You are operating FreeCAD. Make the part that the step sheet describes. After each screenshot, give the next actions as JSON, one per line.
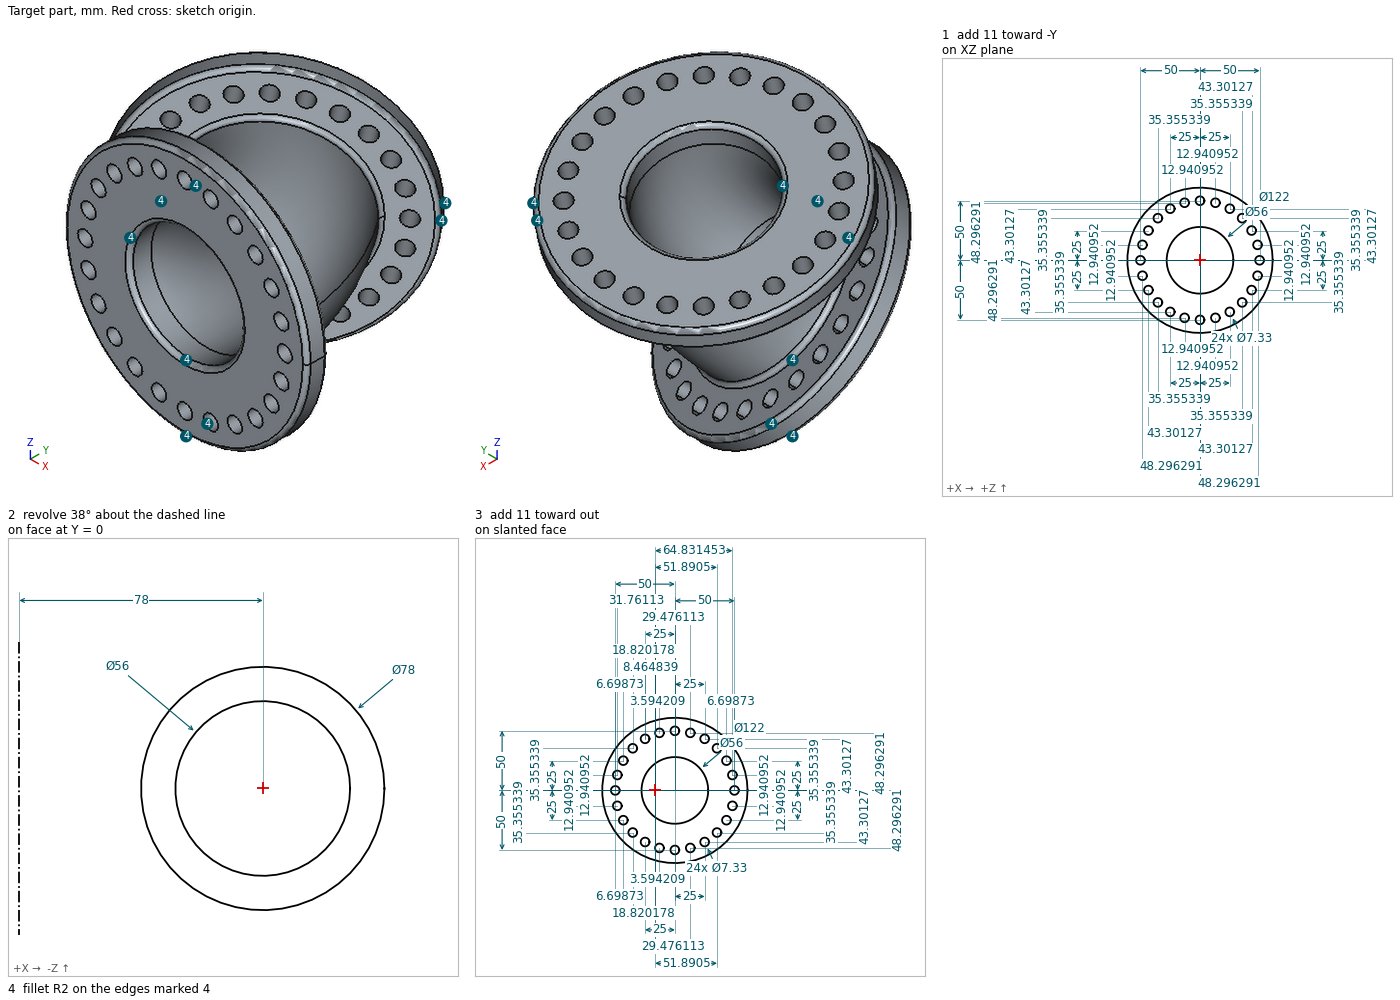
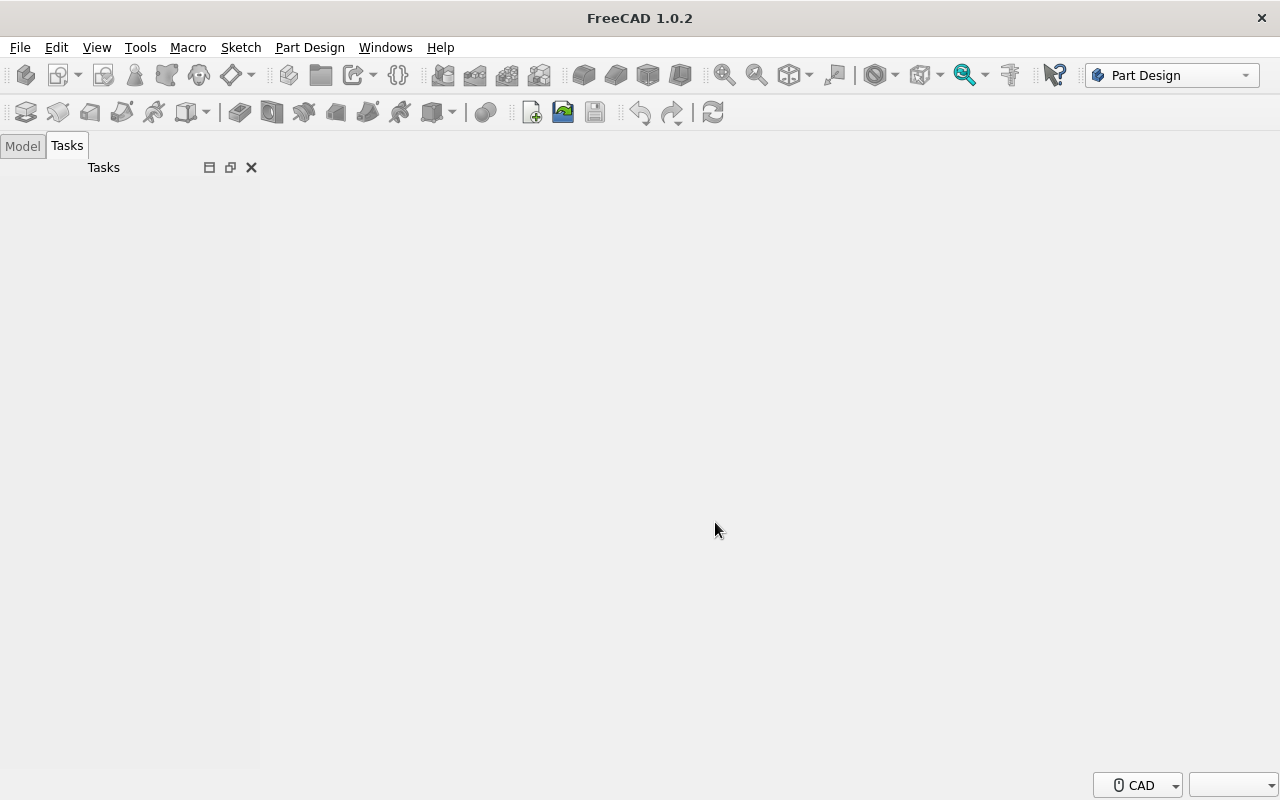
{"action": "left_click", "coordinate": [532, 112]}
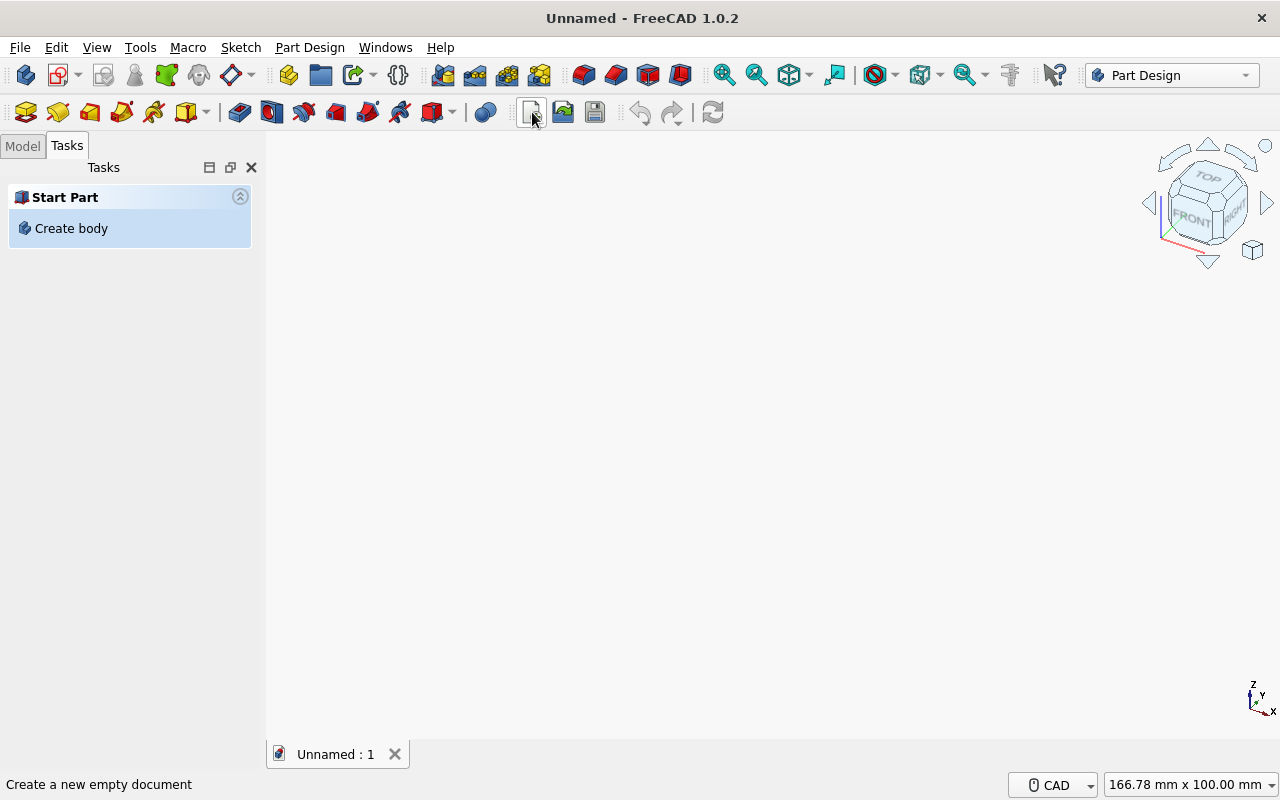
{"action": "left_click", "coordinate": [58, 76]}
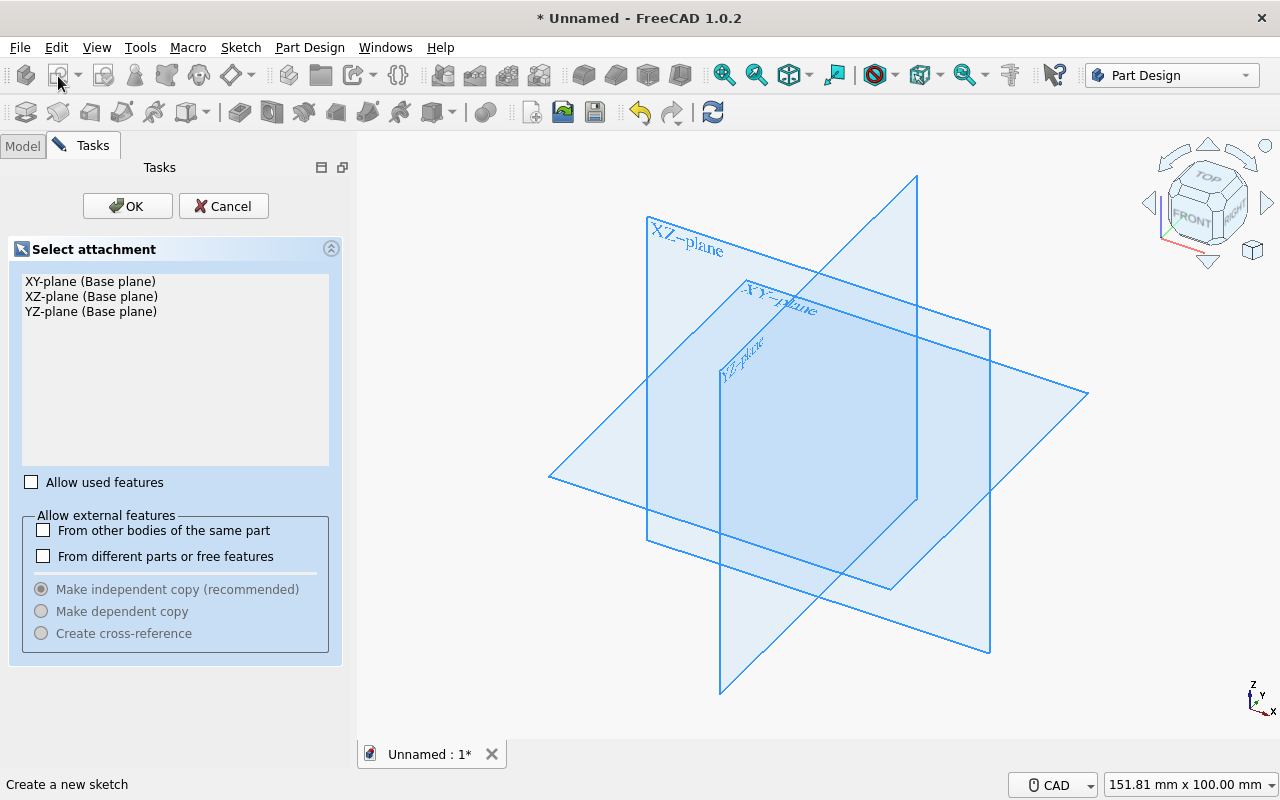
{"action": "left_click", "coordinate": [82, 296]}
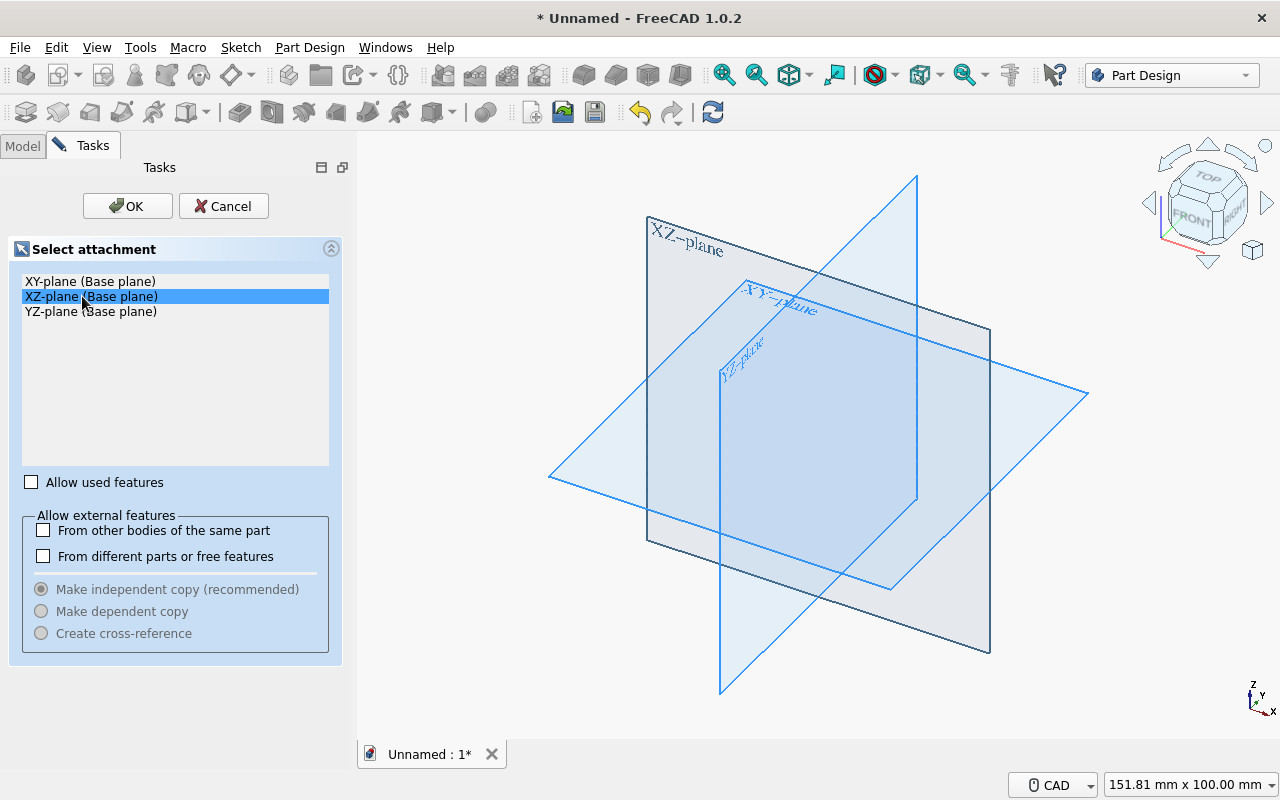
{"action": "left_click", "coordinate": [128, 206]}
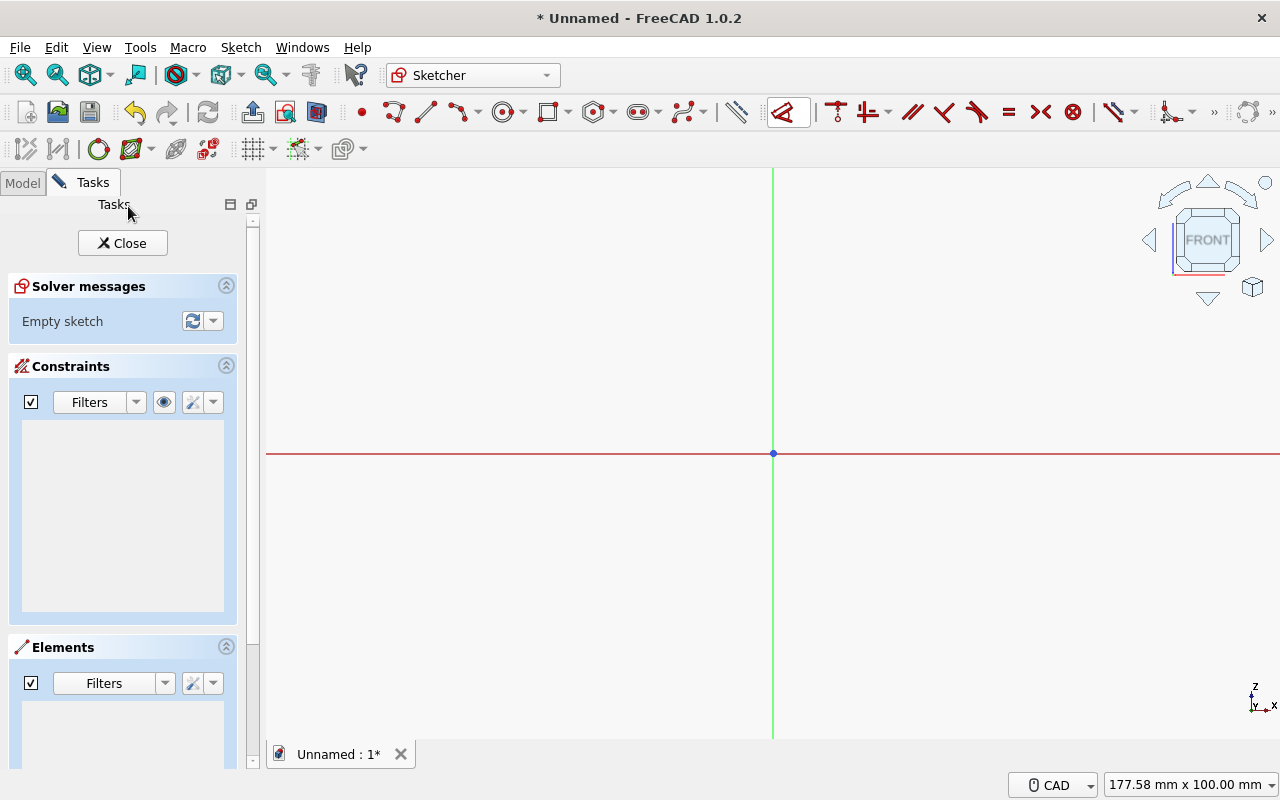
{"action": "scroll", "coordinate": [621, 454], "scroll_direction": "down", "scroll_amount": 3}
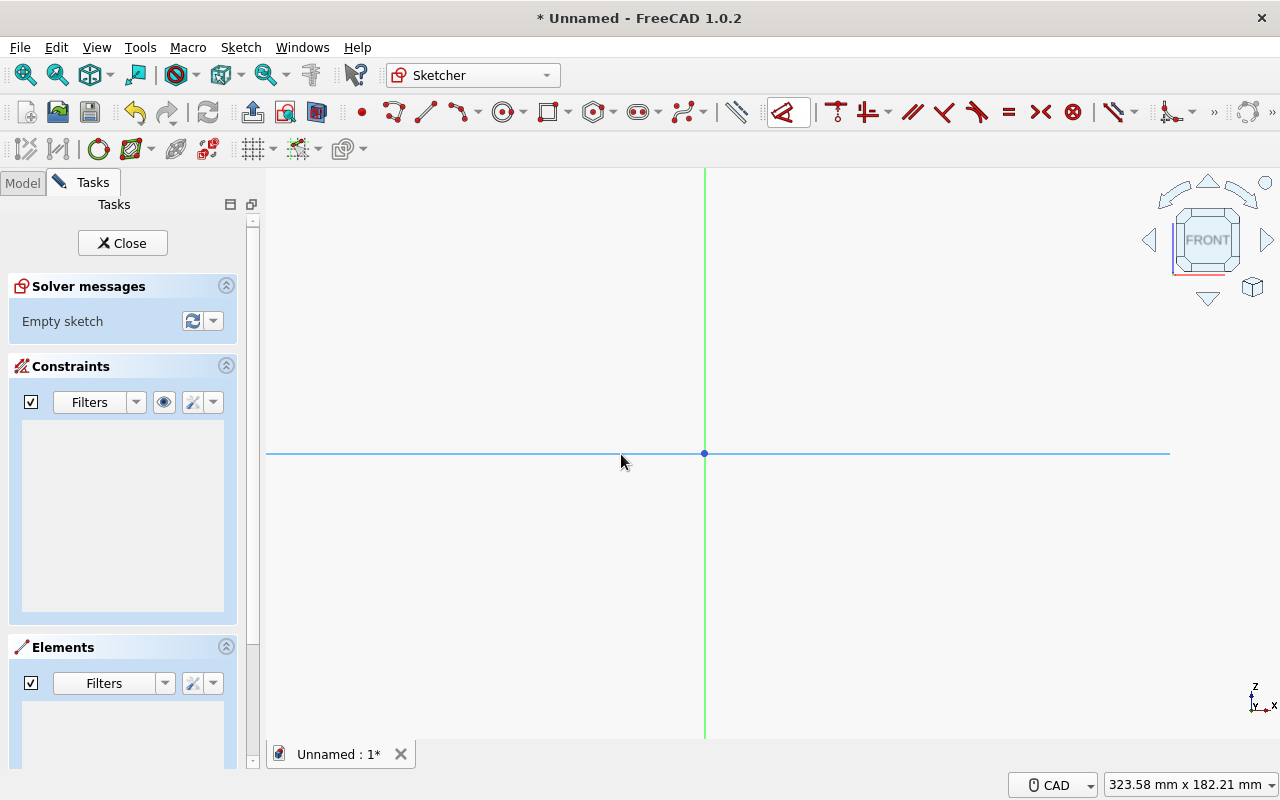
{"action": "left_click", "coordinate": [504, 112]}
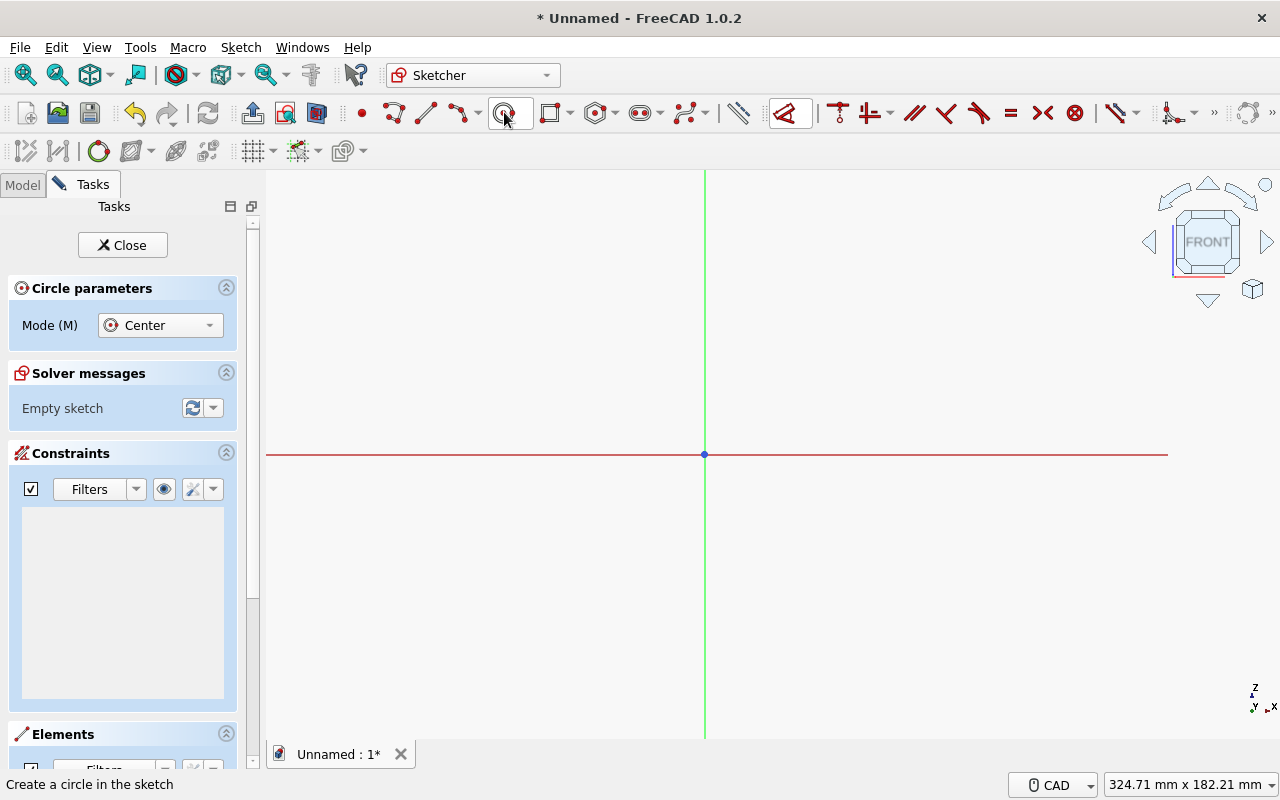
{"action": "left_click", "coordinate": [705, 455]}
{"action": "left_click", "coordinate": [840, 320]}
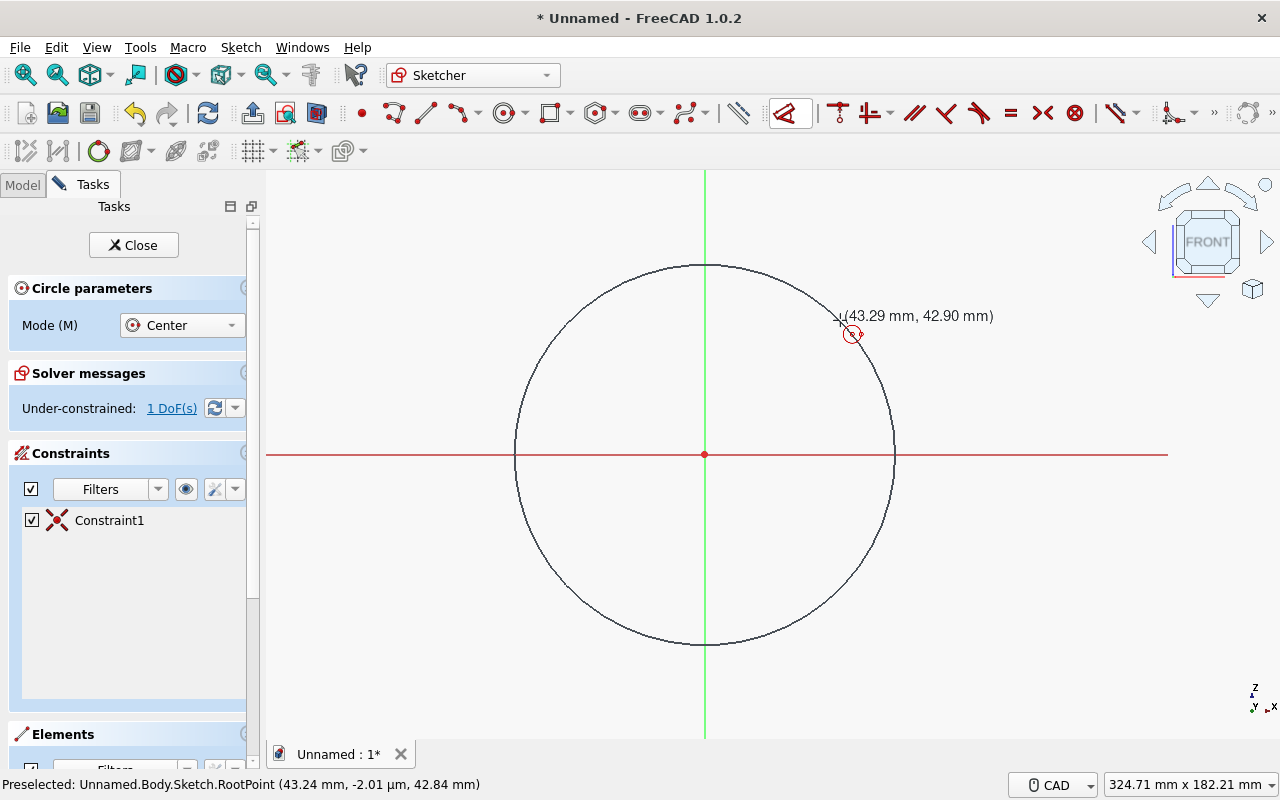
{"action": "scroll", "coordinate": [594, 565], "scroll_direction": "up", "scroll_amount": 4}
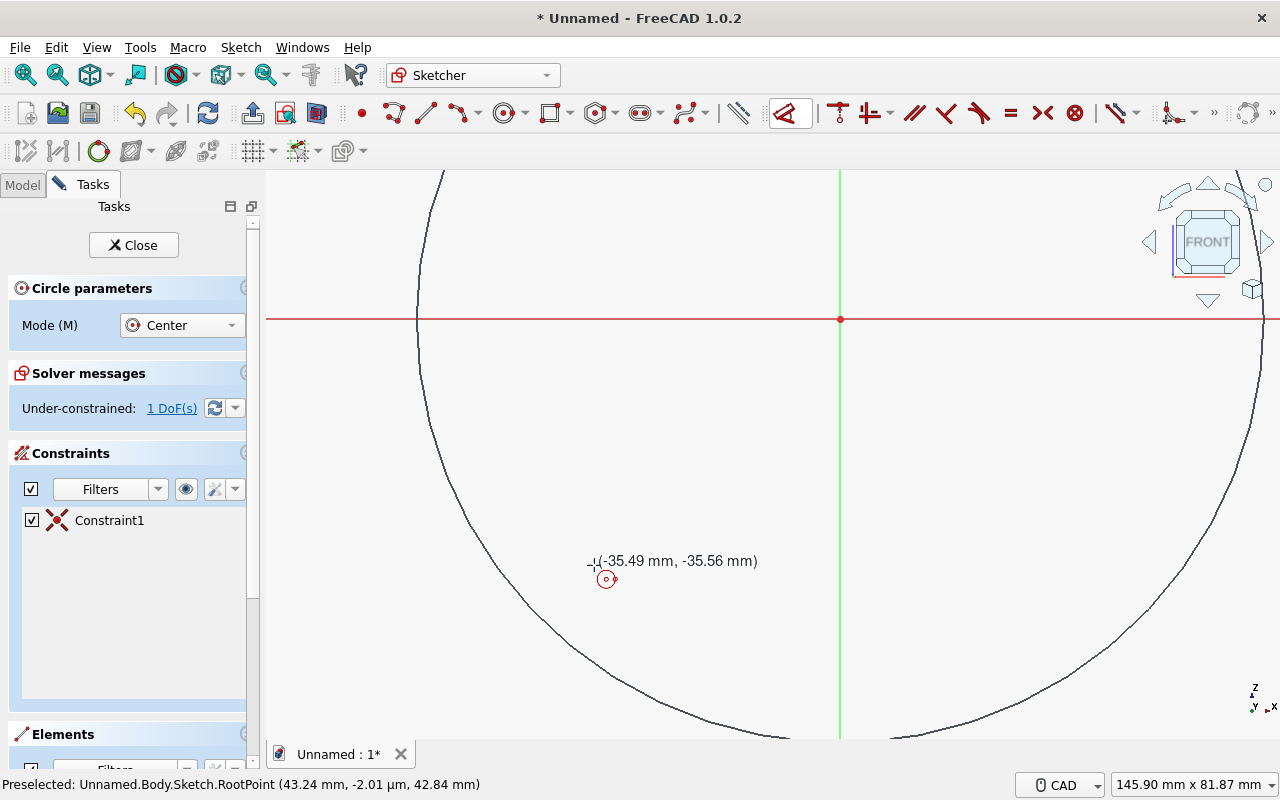
{"action": "left_click", "coordinate": [595, 565]}
{"action": "left_click", "coordinate": [613, 547]}